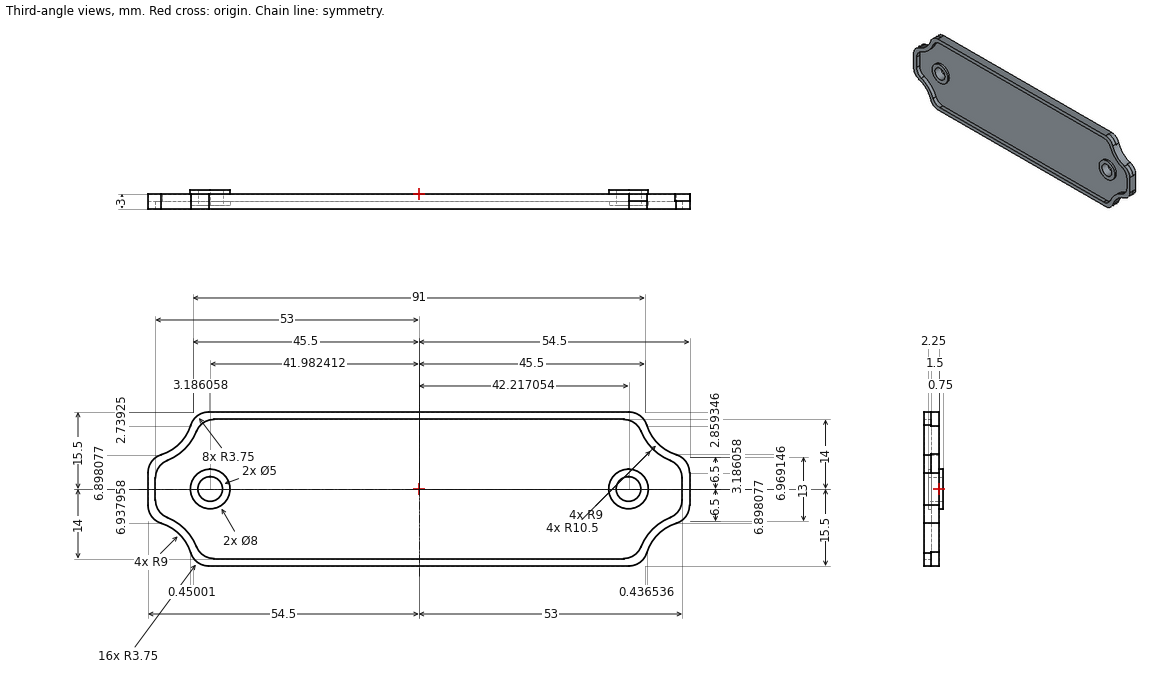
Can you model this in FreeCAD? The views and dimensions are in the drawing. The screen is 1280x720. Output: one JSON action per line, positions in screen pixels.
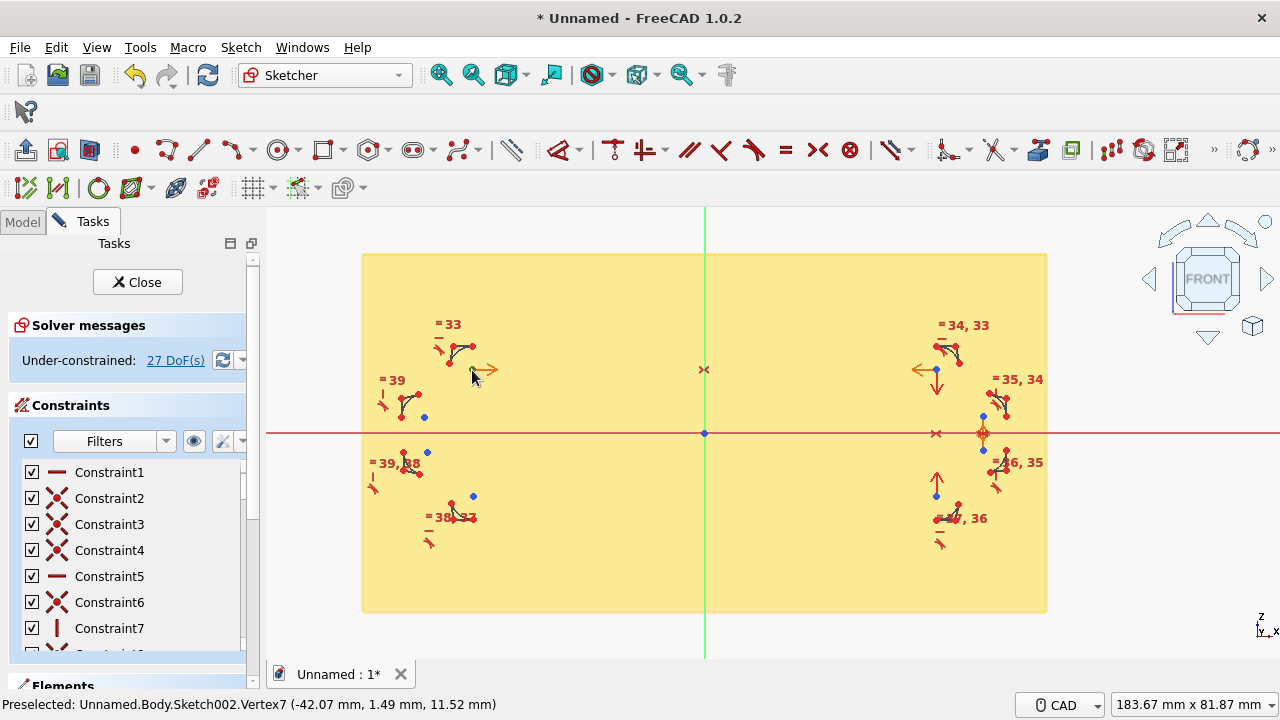
{"action": "left_click", "coordinate": [474, 496]}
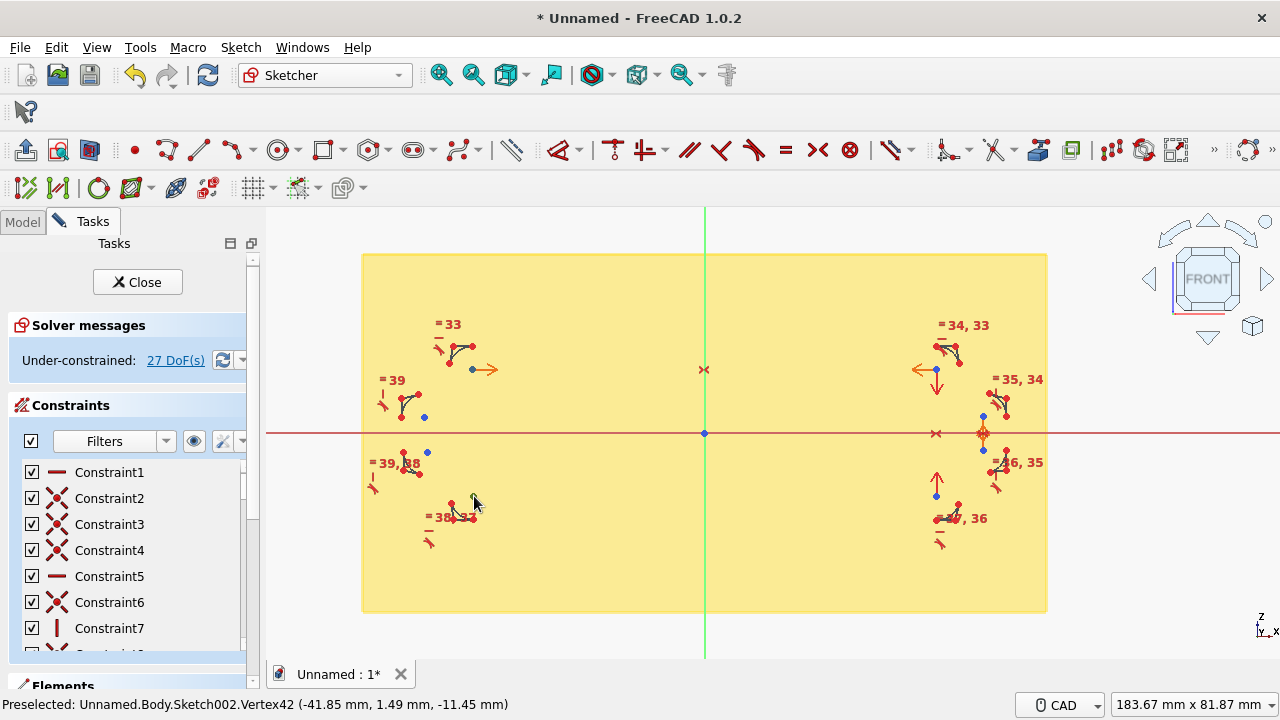
{"action": "left_click", "coordinate": [353, 433]}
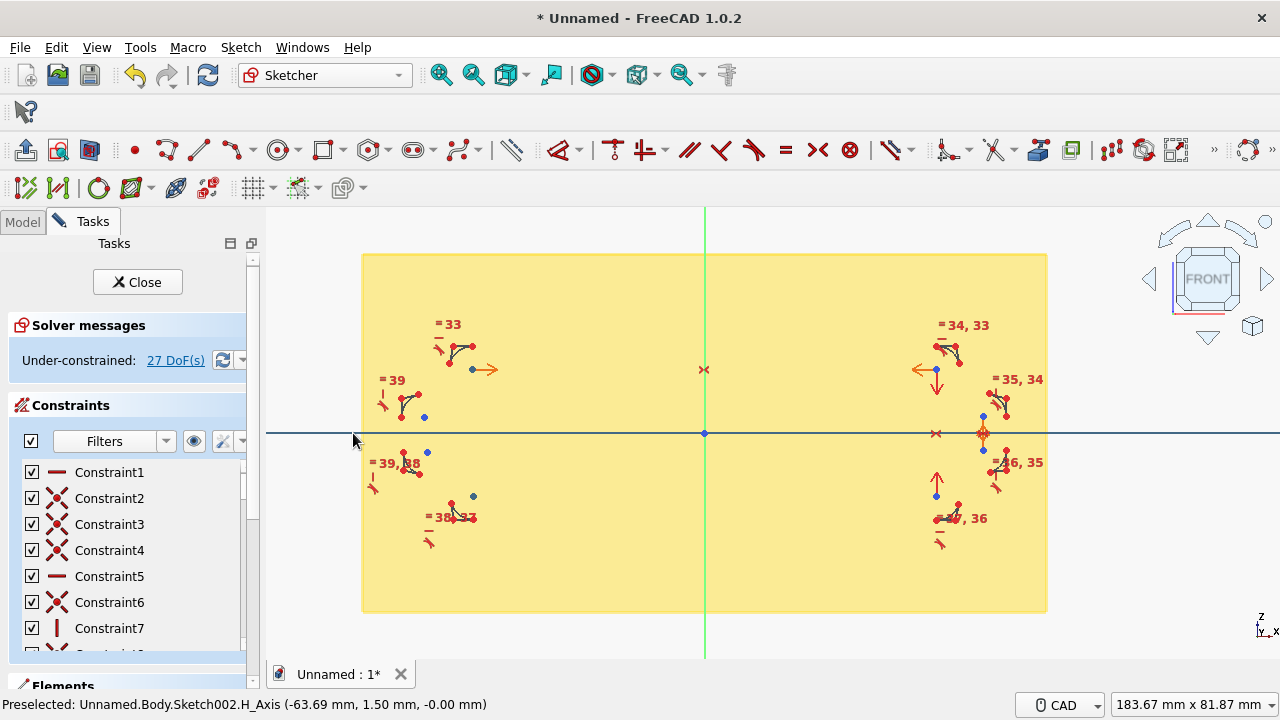
{"action": "left_click", "coordinate": [818, 150]}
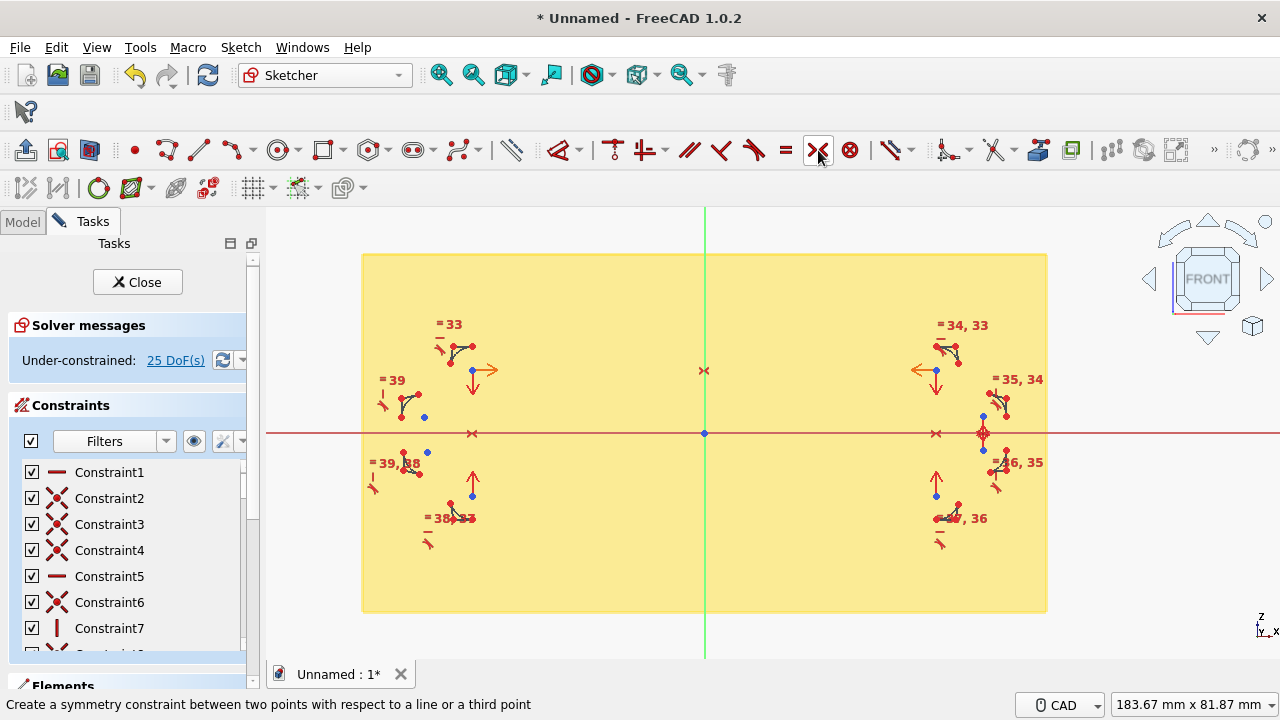
{"action": "left_click", "coordinate": [983, 450]}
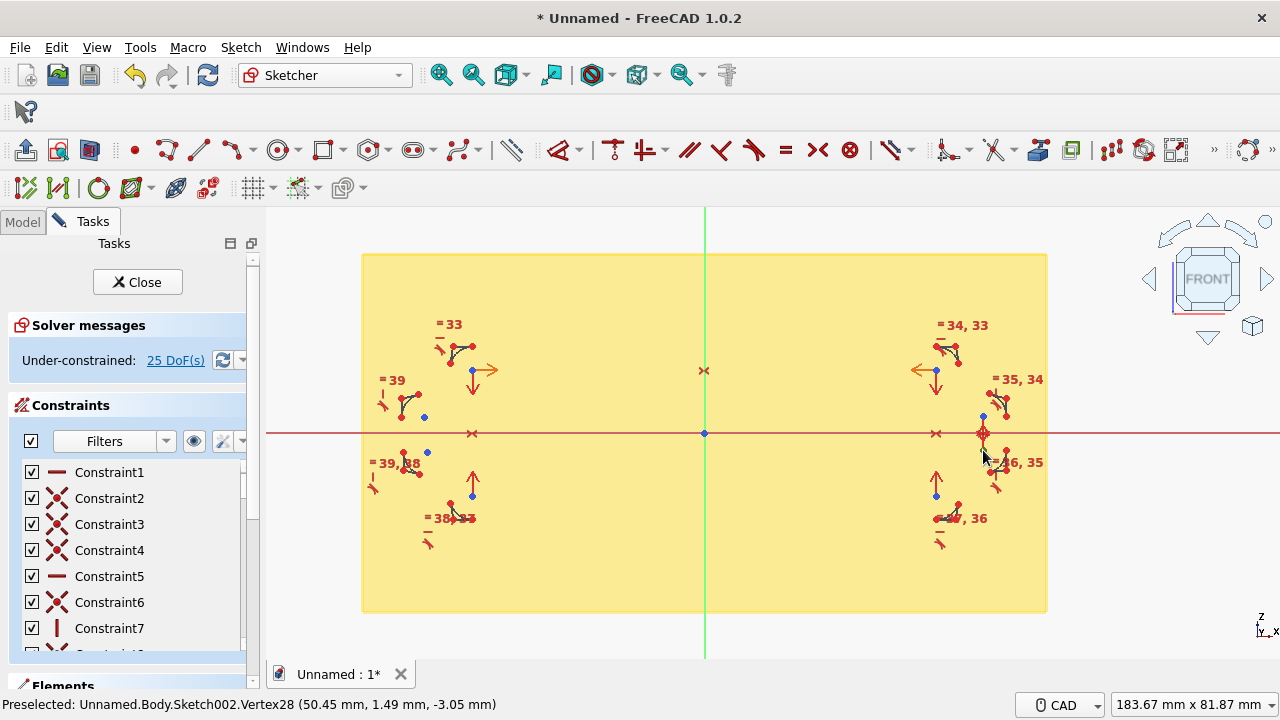
{"action": "left_click", "coordinate": [427, 452]}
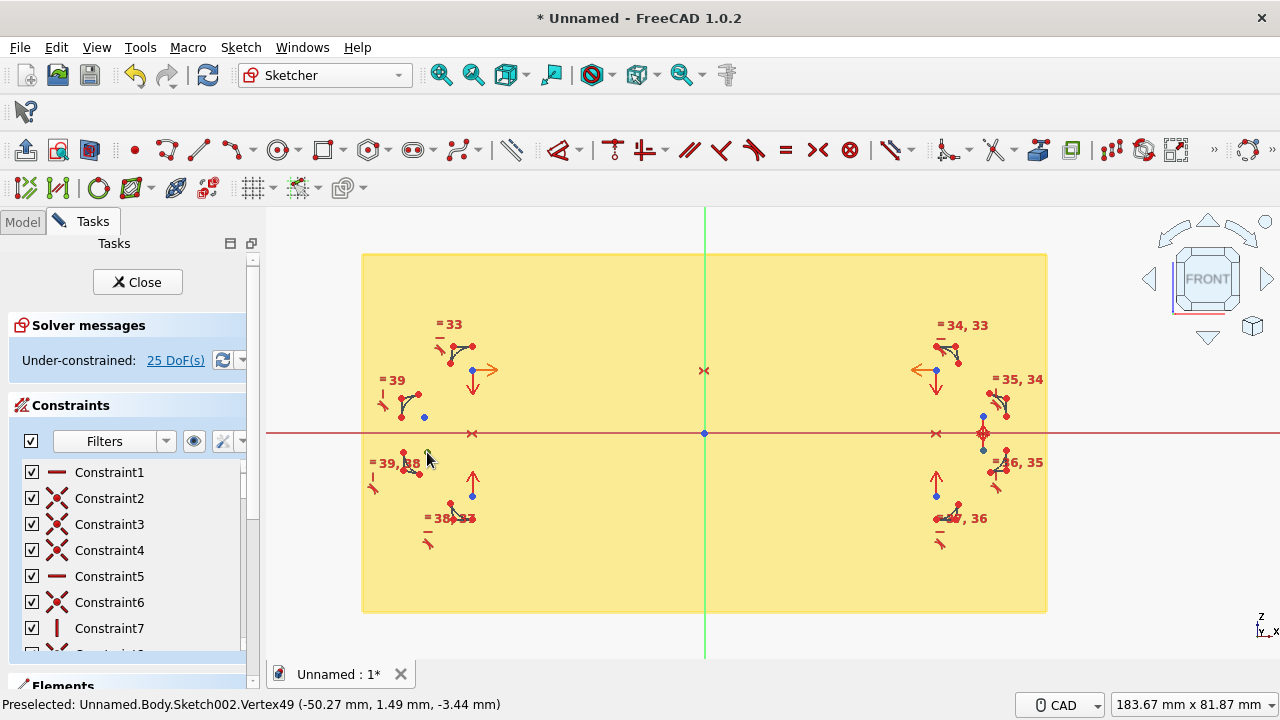
{"action": "left_click", "coordinate": [705, 603]}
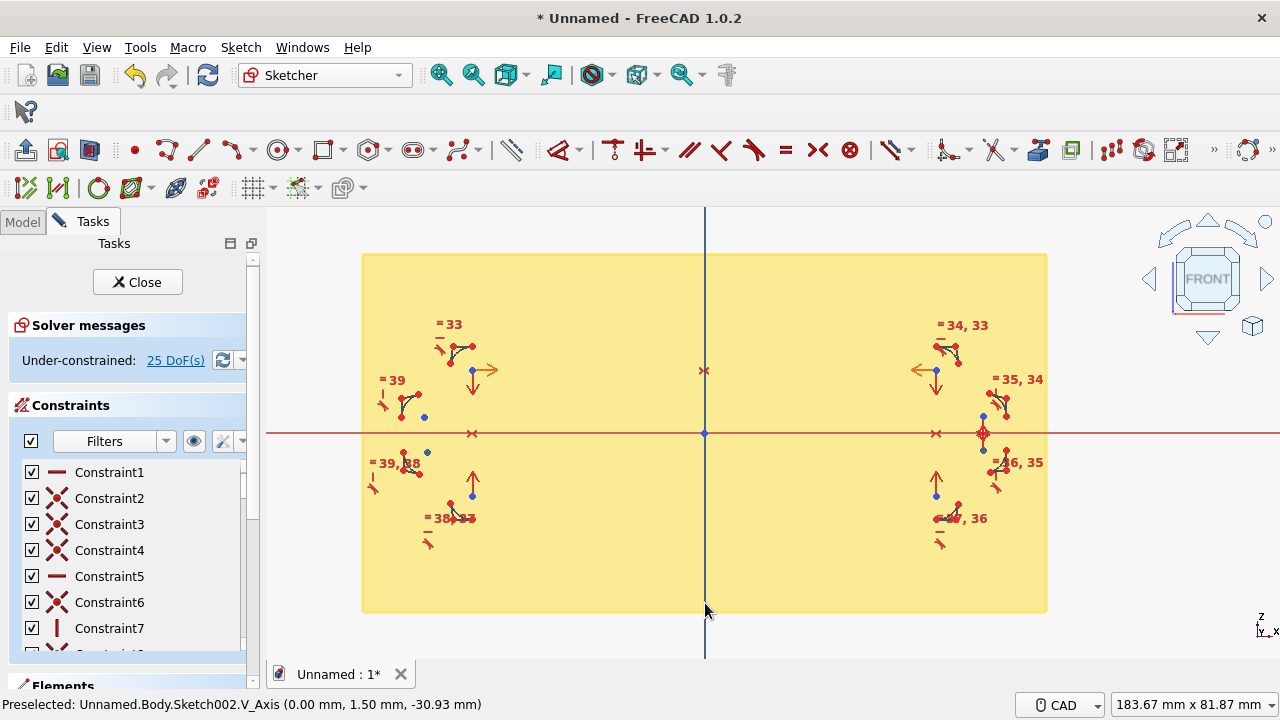
{"action": "left_click", "coordinate": [818, 150]}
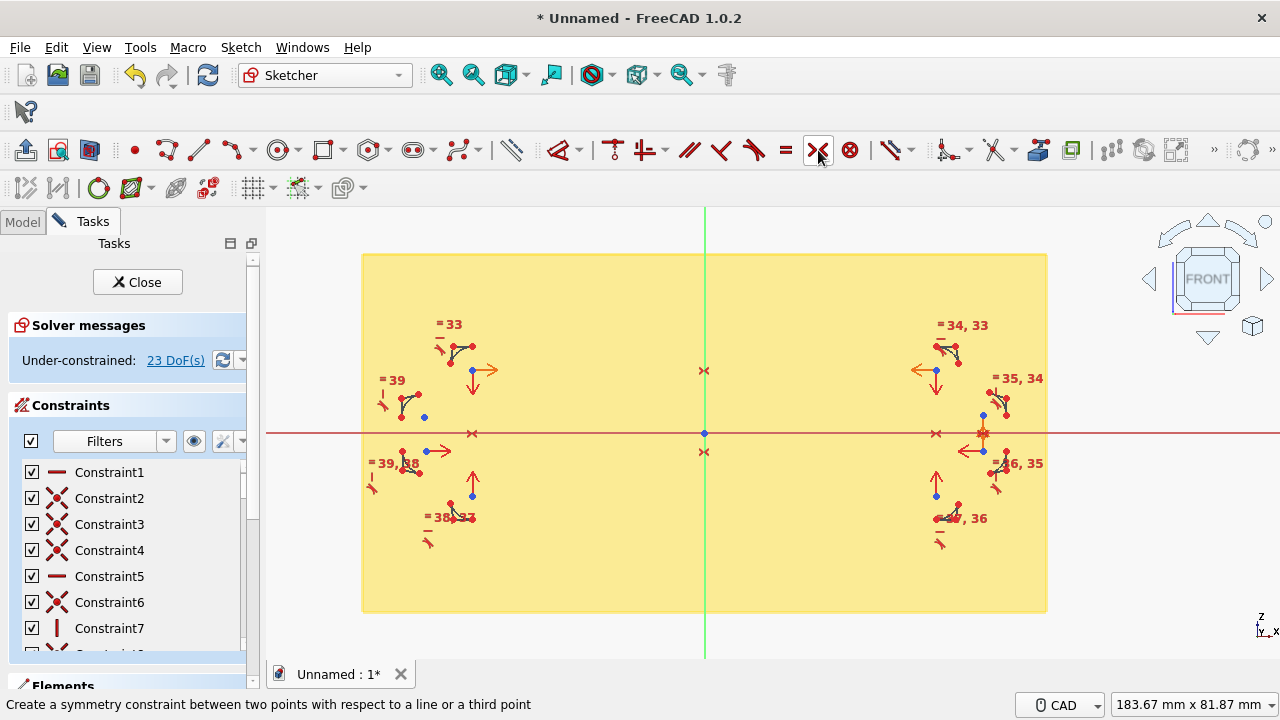
{"action": "left_click", "coordinate": [983, 415]}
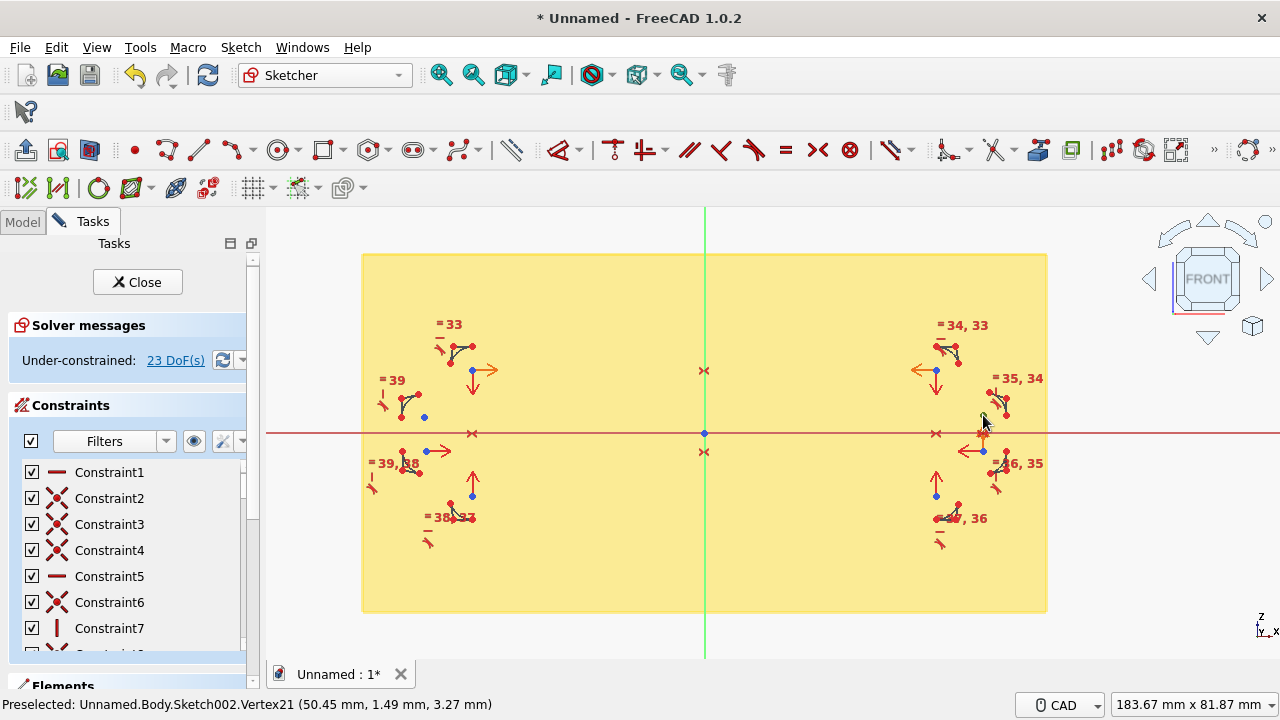
{"action": "left_click", "coordinate": [425, 417]}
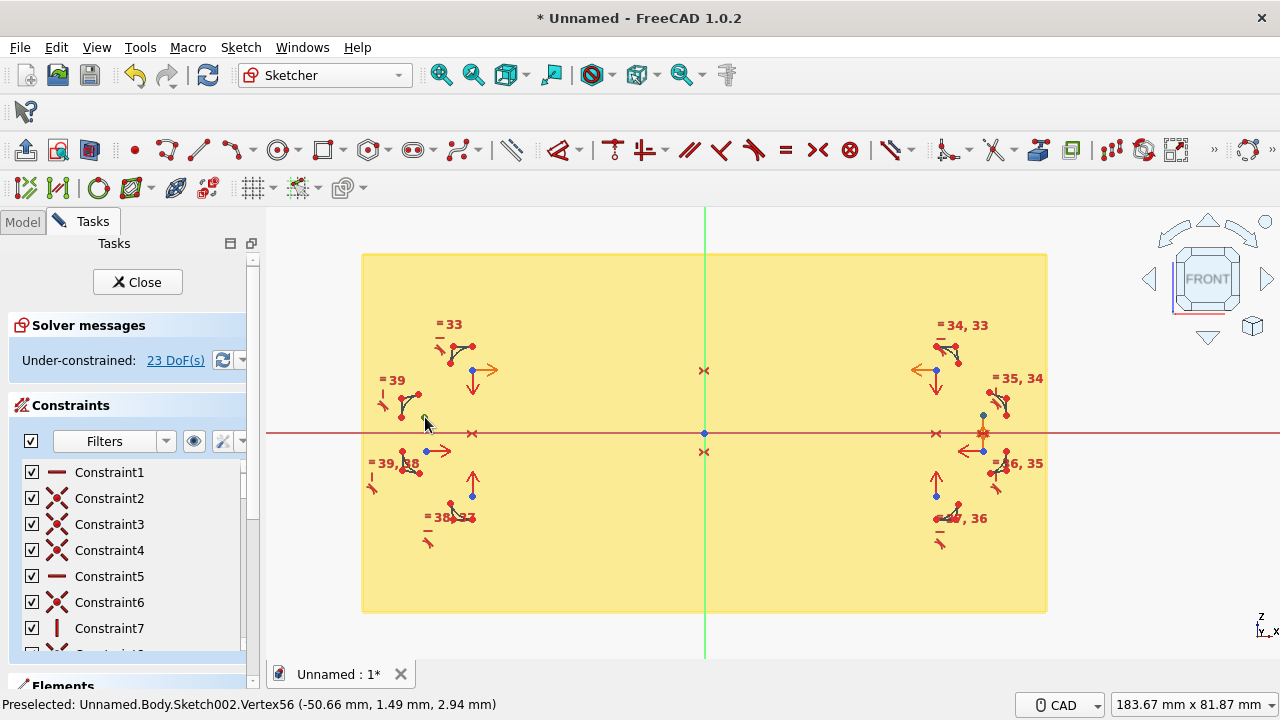
{"action": "left_click", "coordinate": [705, 603]}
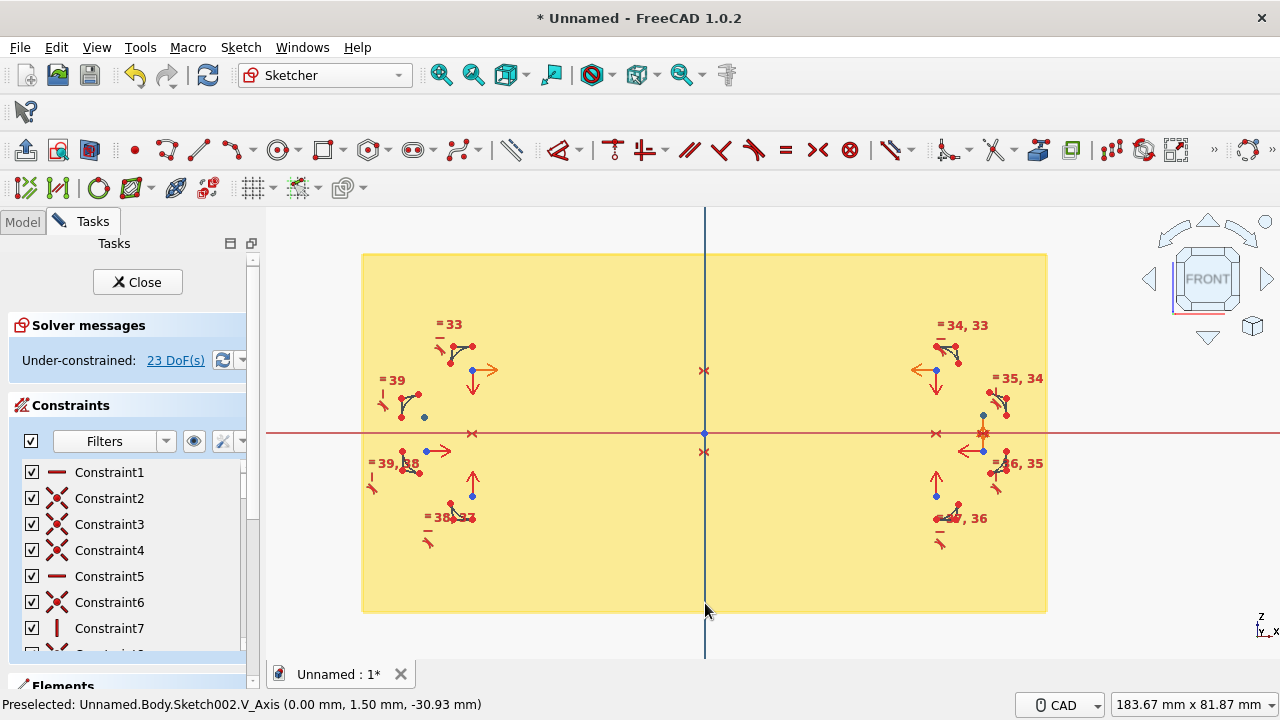
{"action": "left_click", "coordinate": [818, 150]}